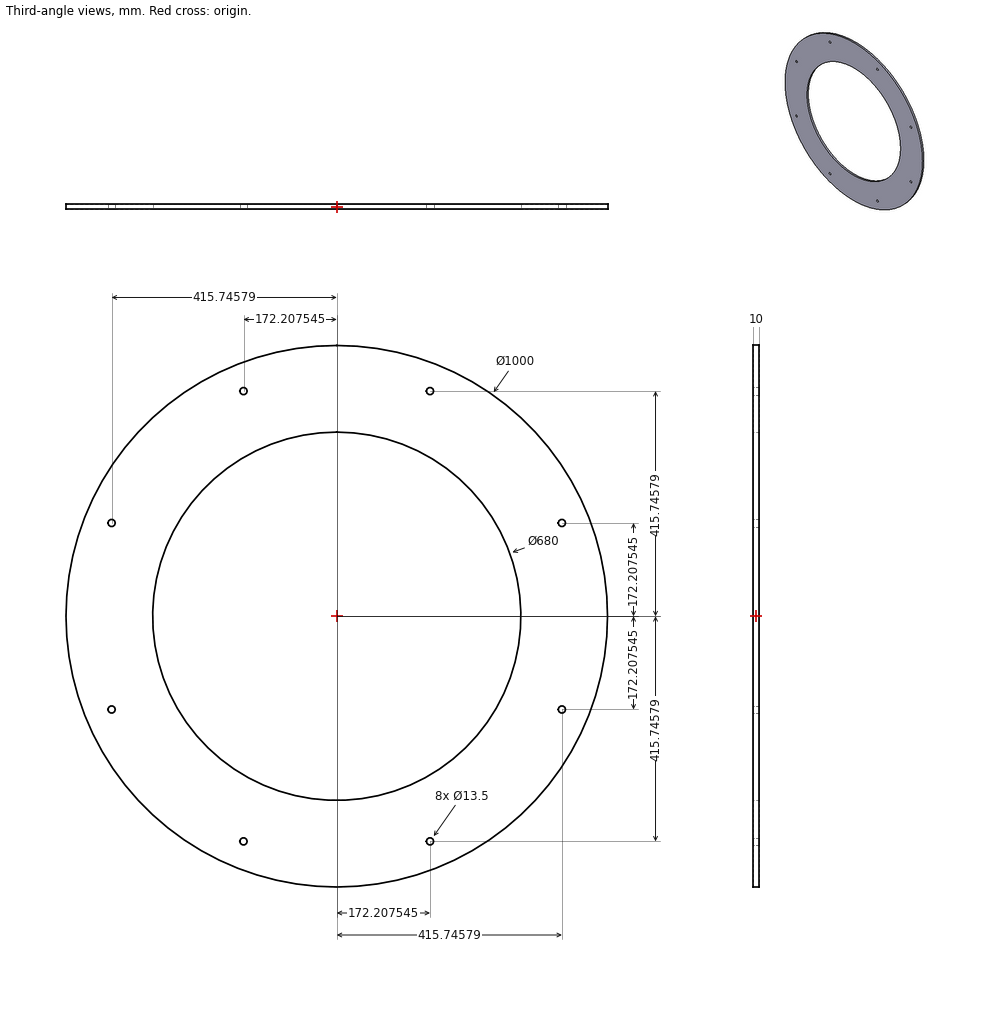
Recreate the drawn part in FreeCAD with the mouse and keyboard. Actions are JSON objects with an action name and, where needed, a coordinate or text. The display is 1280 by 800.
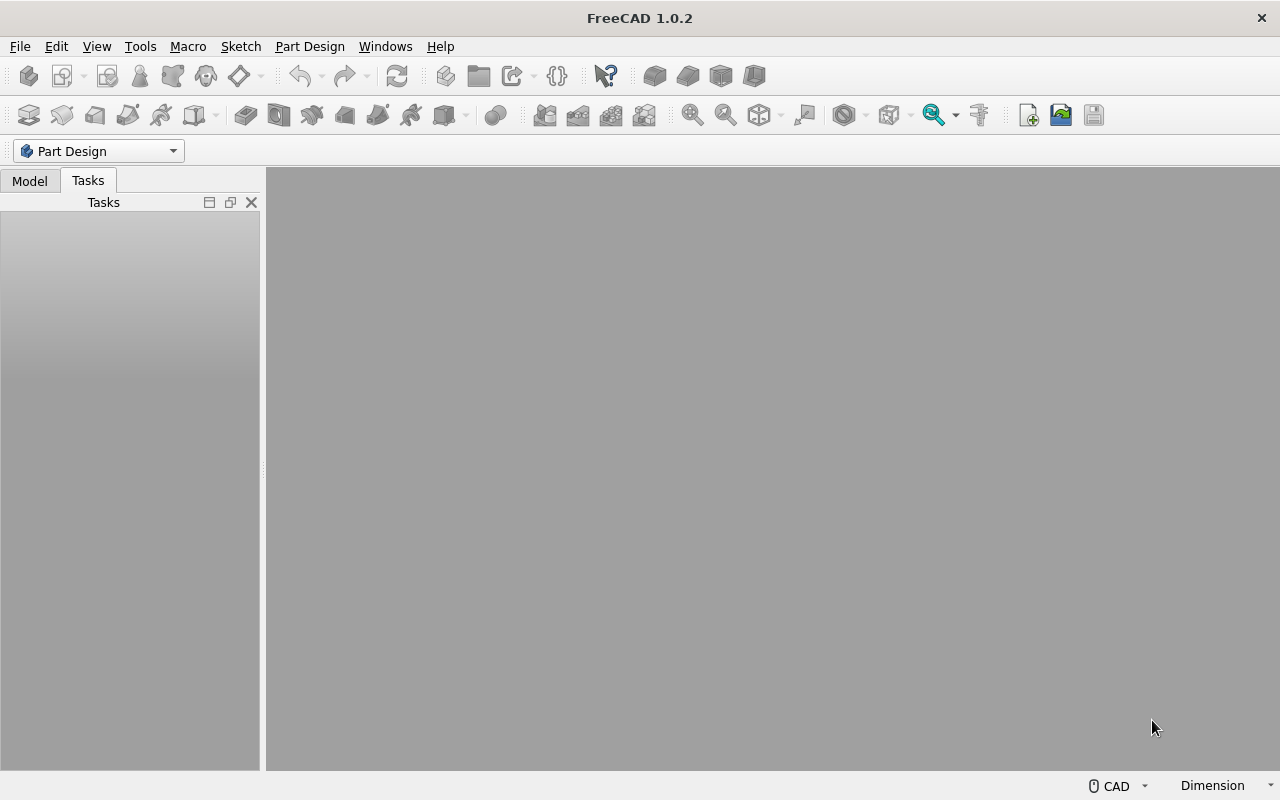
{"action": "key", "text": "ctrl+n"}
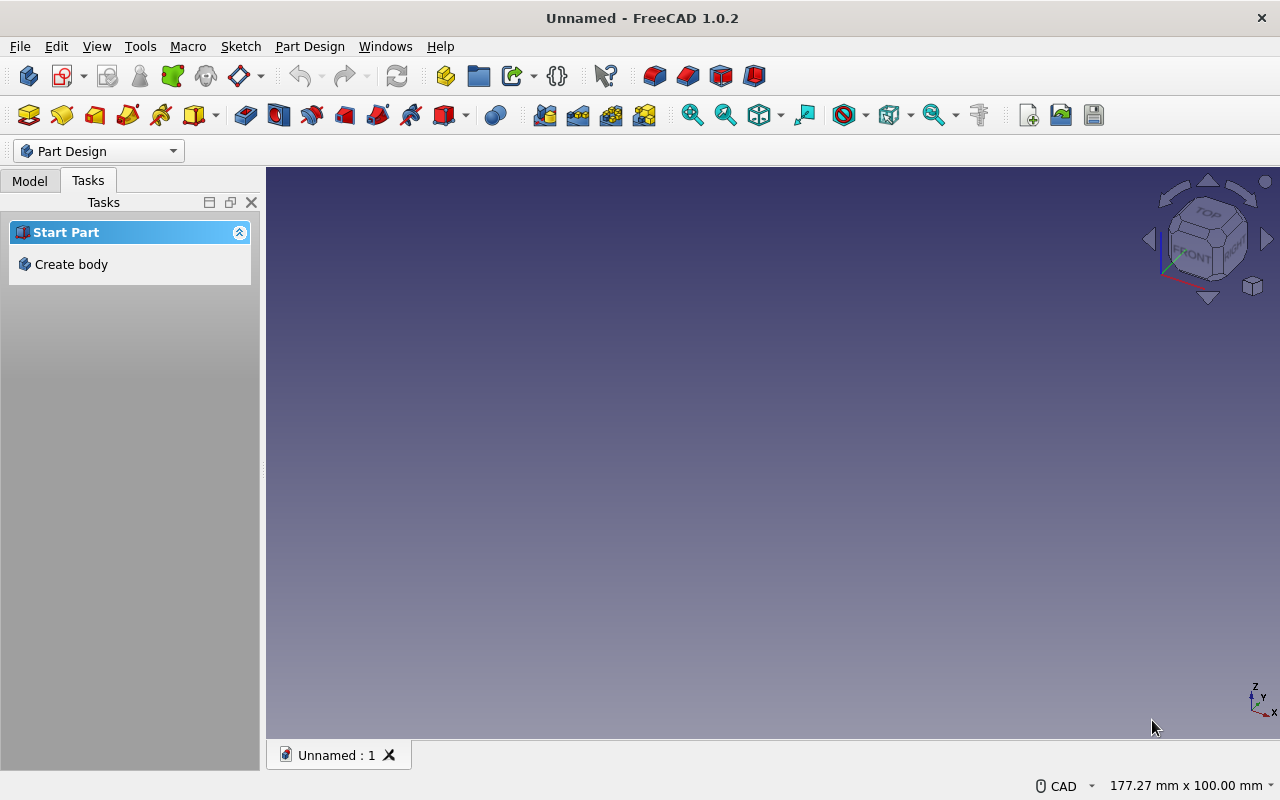
{"action": "left_click", "coordinate": [62, 76]}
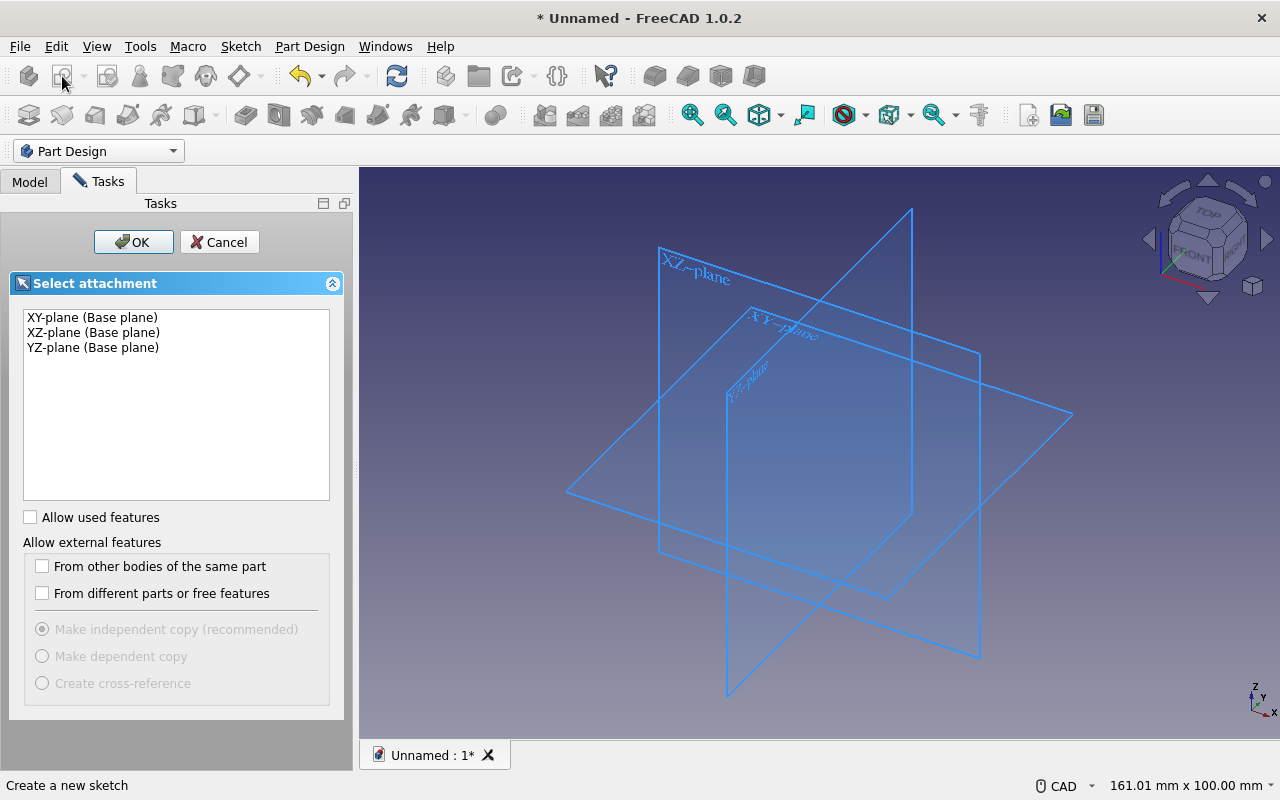
{"action": "left_click", "coordinate": [84, 332]}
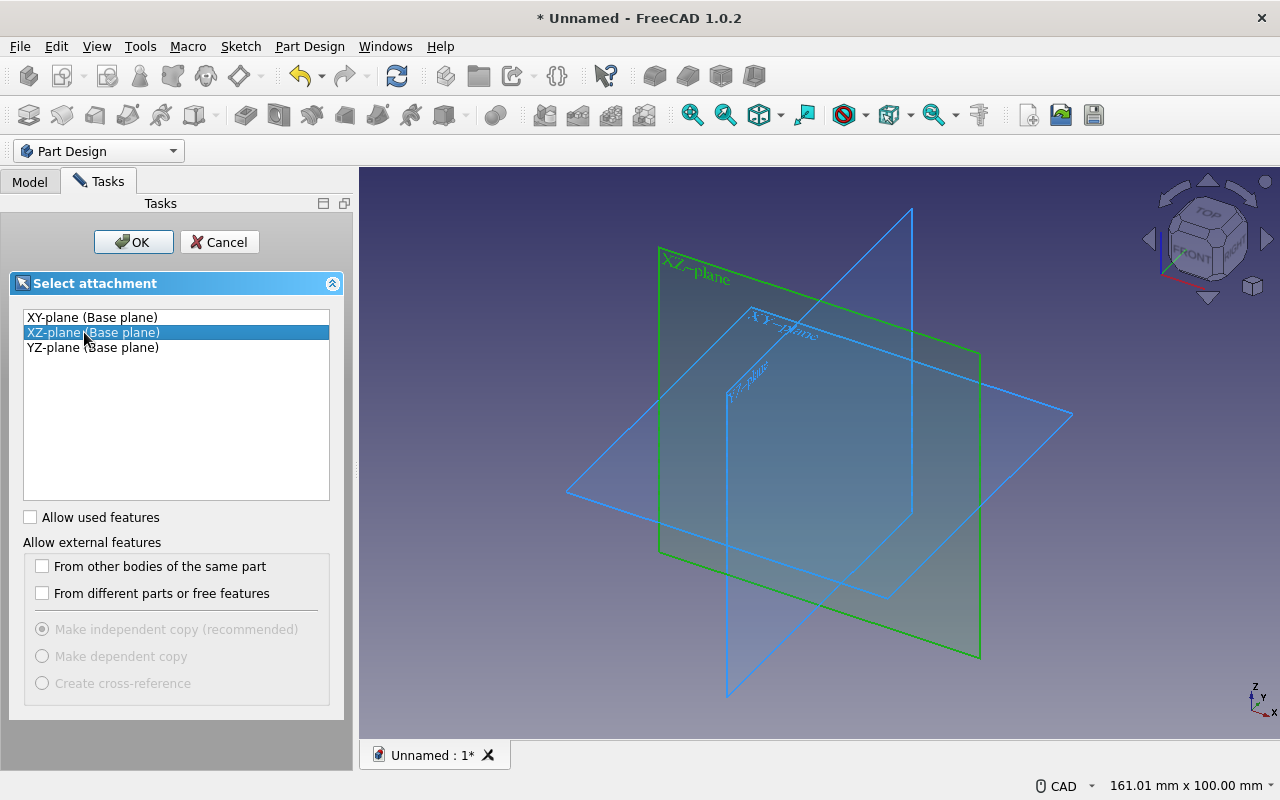
{"action": "left_click", "coordinate": [134, 242]}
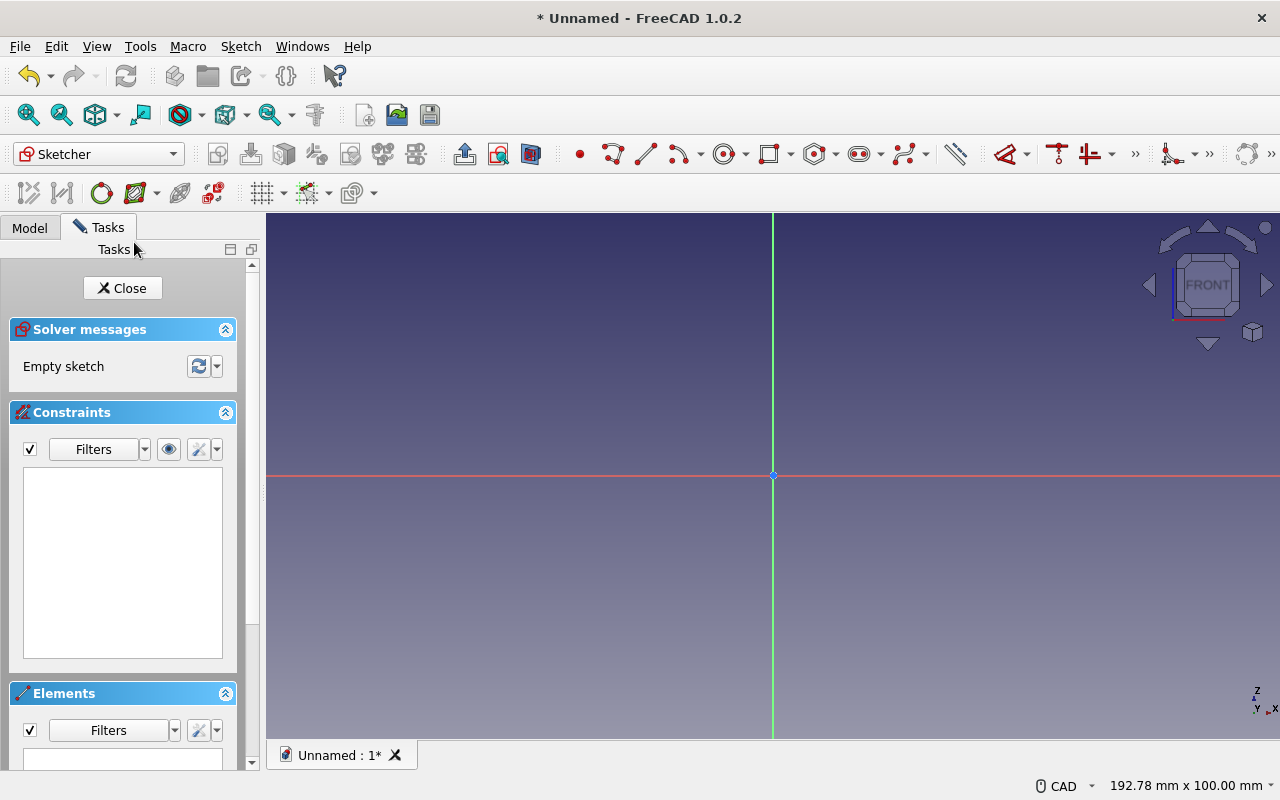
{"action": "scroll", "coordinate": [700, 476], "scroll_direction": "down", "scroll_amount": 14}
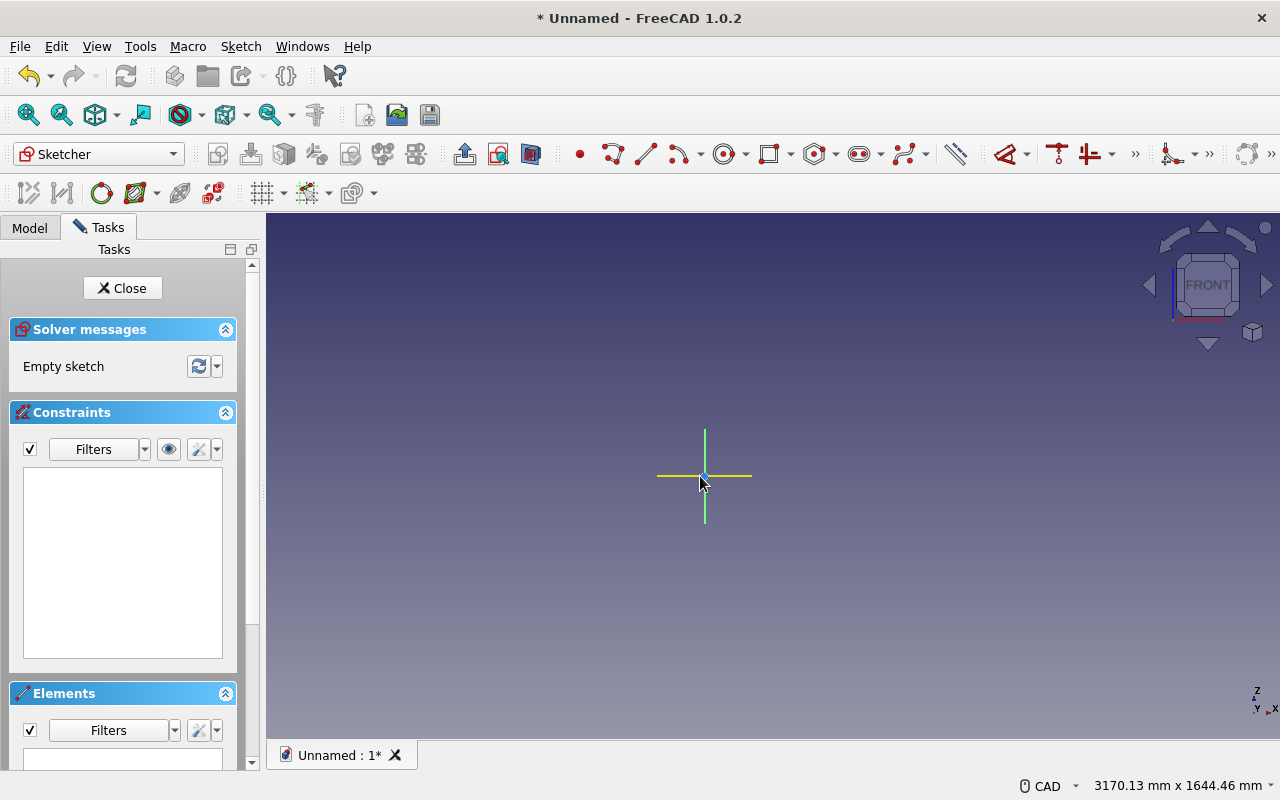
{"action": "key", "text": "g c"}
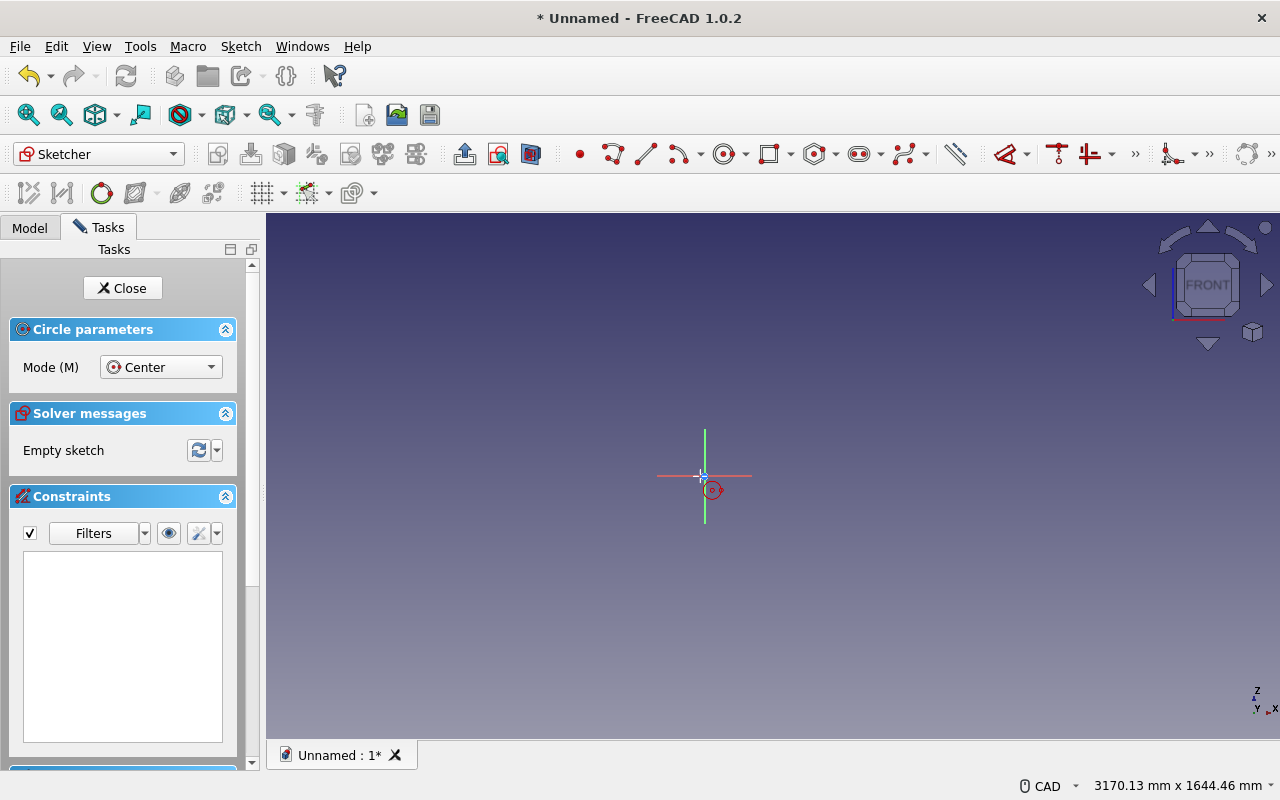
{"action": "left_click", "coordinate": [705, 476]}
{"action": "mouse_move", "coordinate": [818, 363]}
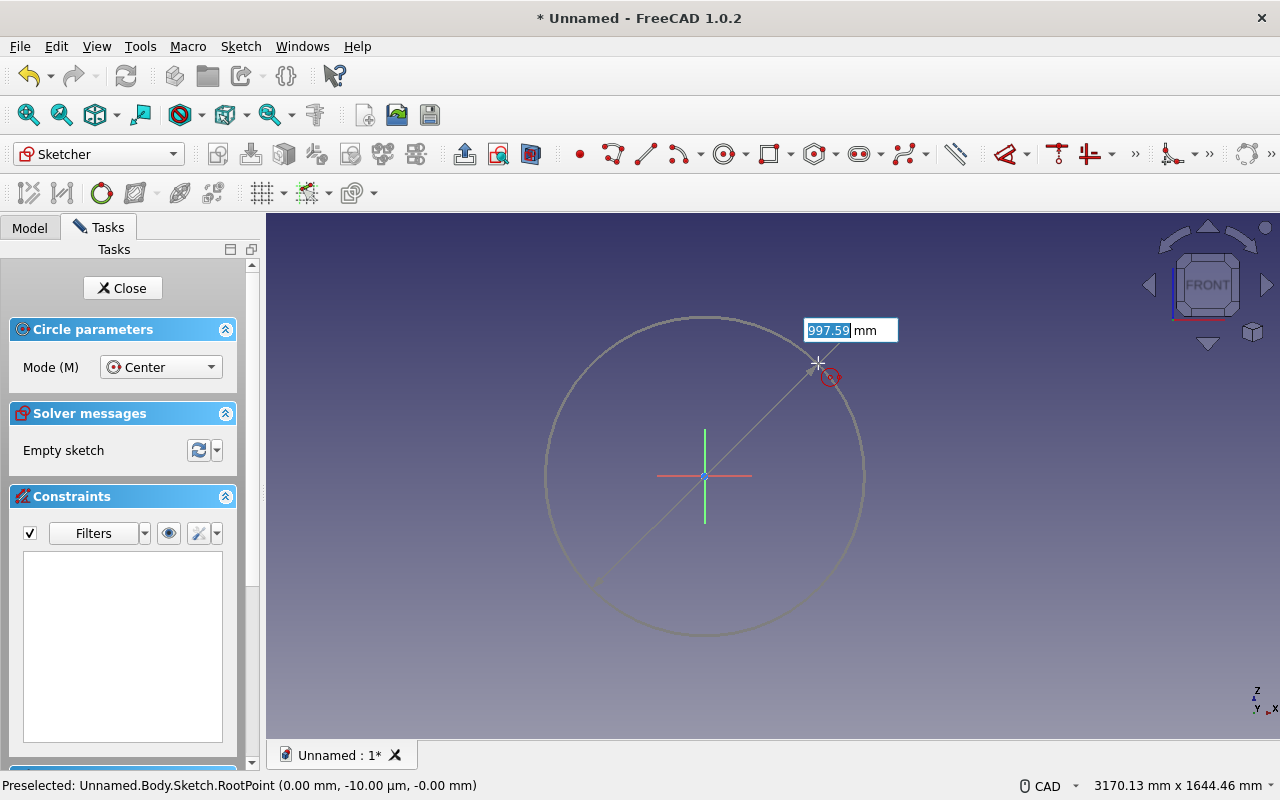
{"action": "type", "text": "1000"}
{"action": "key", "text": "Return"}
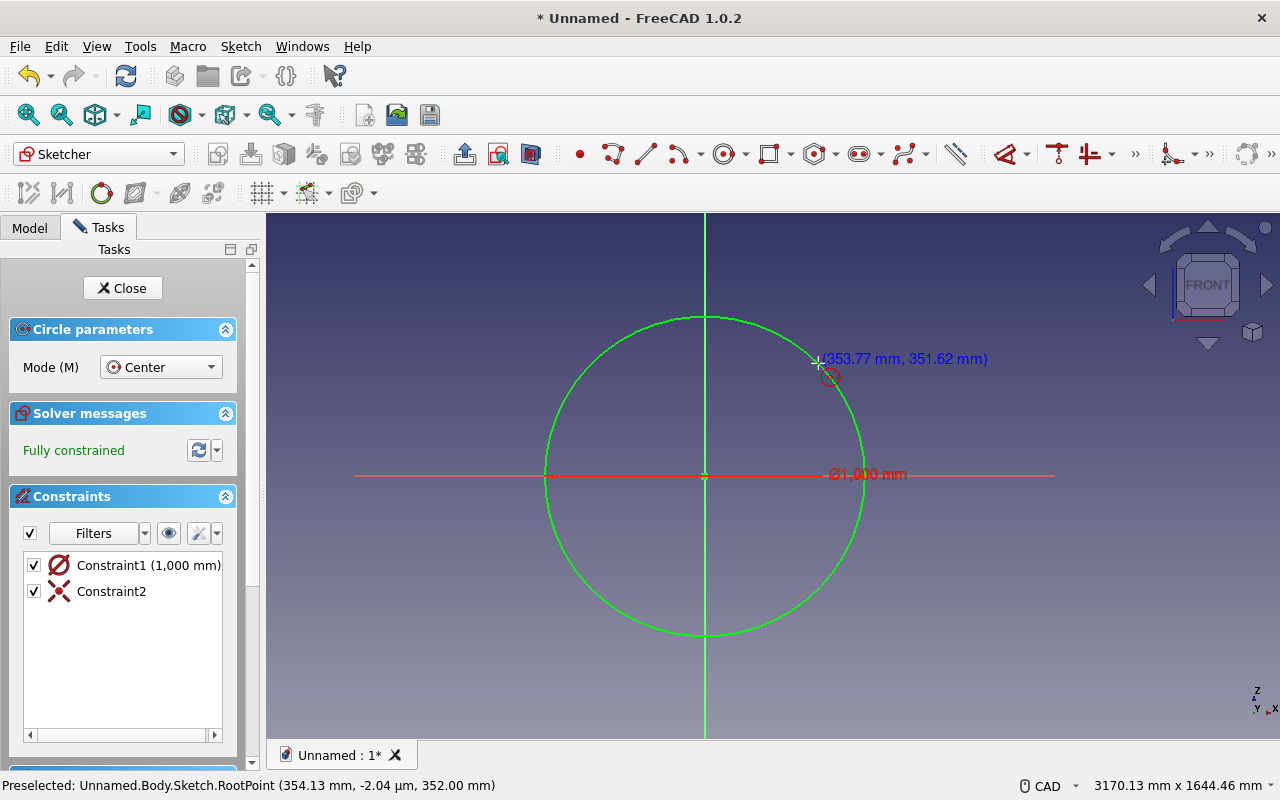
{"action": "left_click", "coordinate": [705, 476]}
{"action": "mouse_move", "coordinate": [782, 400]}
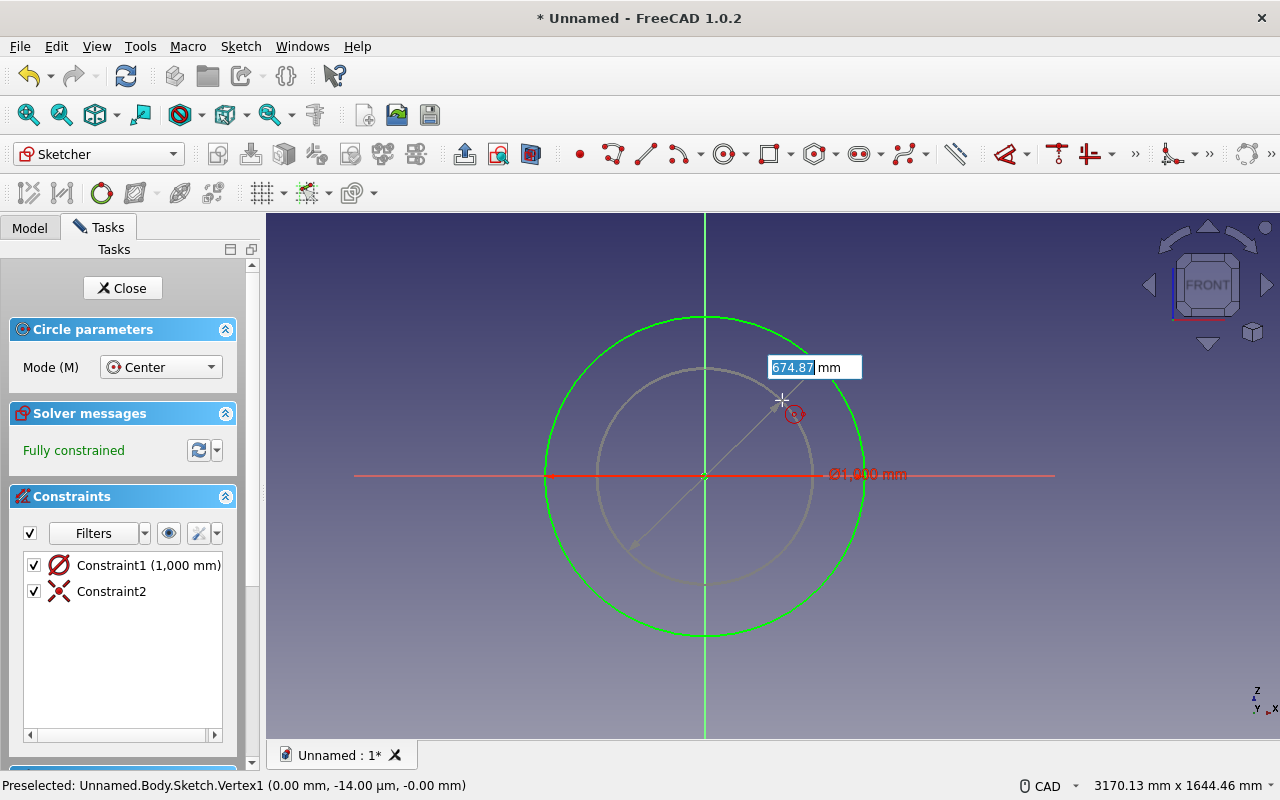
{"action": "type", "text": "680"}
{"action": "key", "text": "Return"}
{"action": "key", "text": "Escape"}